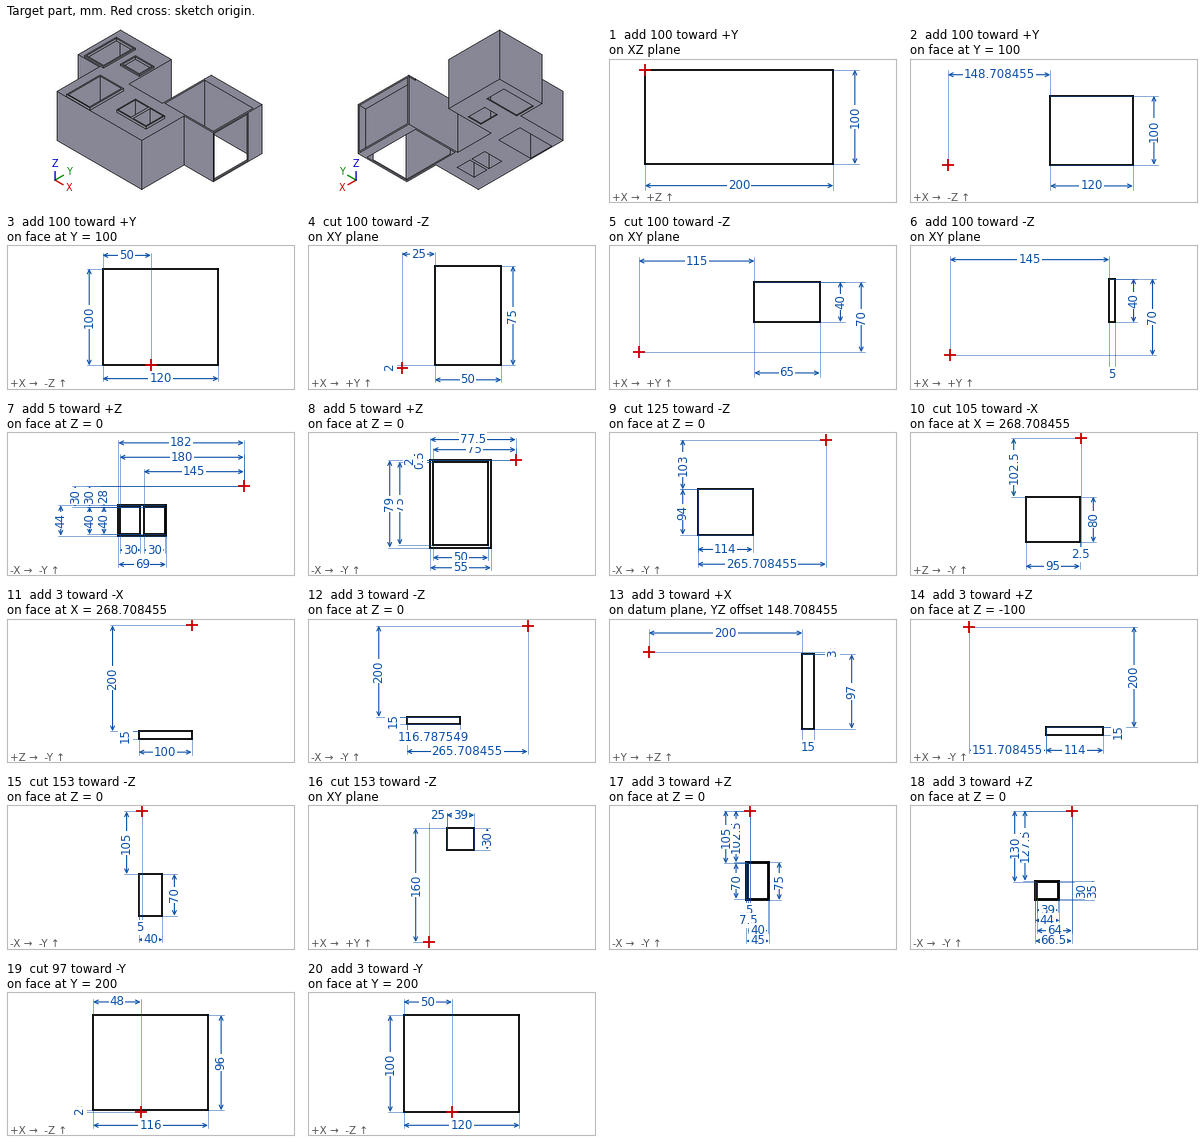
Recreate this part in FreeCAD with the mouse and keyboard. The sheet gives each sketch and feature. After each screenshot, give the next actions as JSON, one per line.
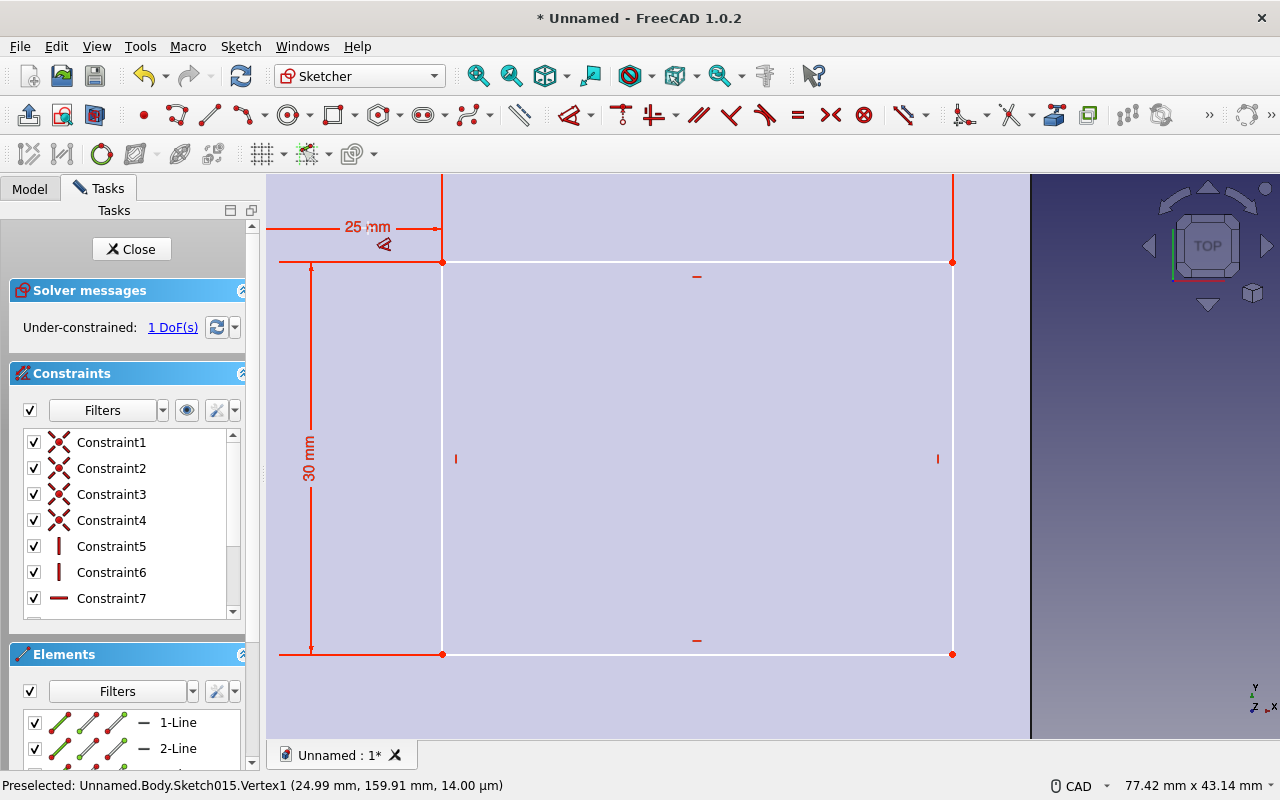
{"action": "left_click", "coordinate": [442, 262]}
{"action": "left_click", "coordinate": [476, 487]}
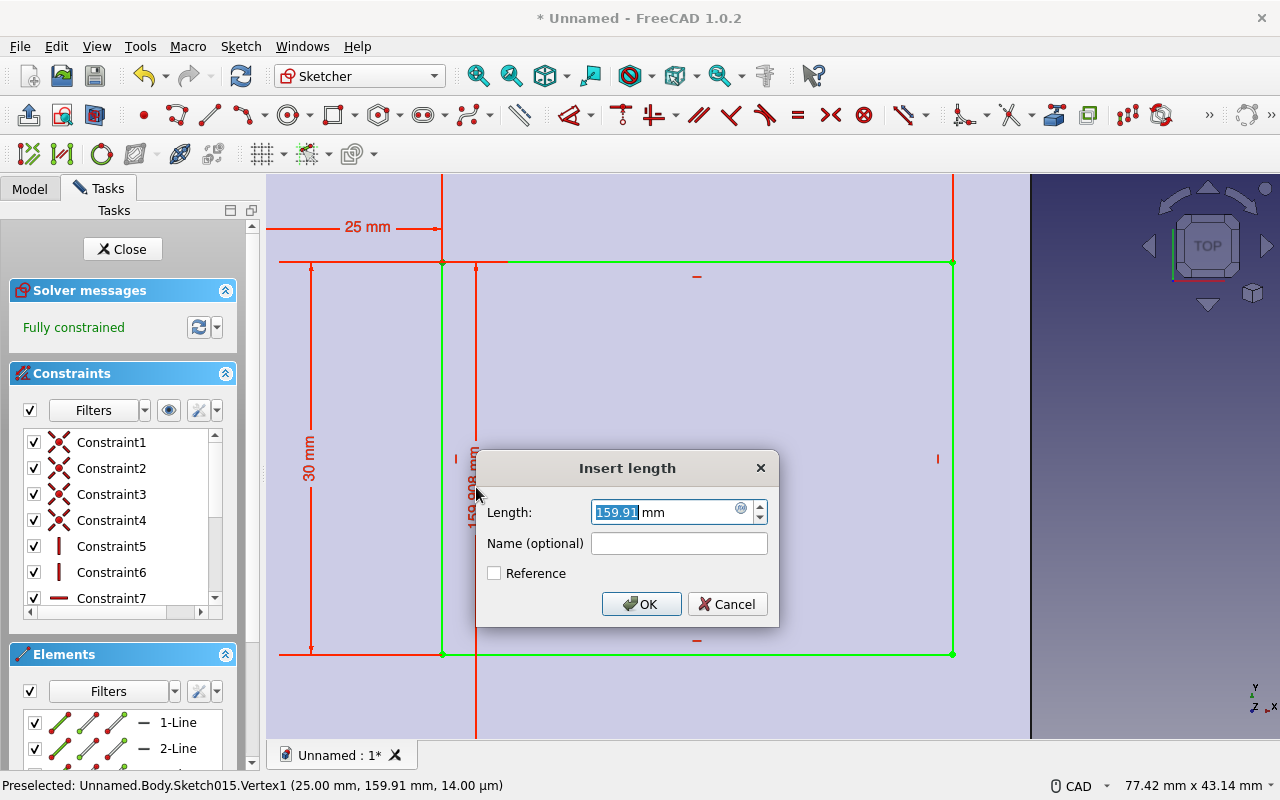
{"action": "type", "text": "160"}
{"action": "key", "text": "Return"}
{"action": "key", "text": "Escape"}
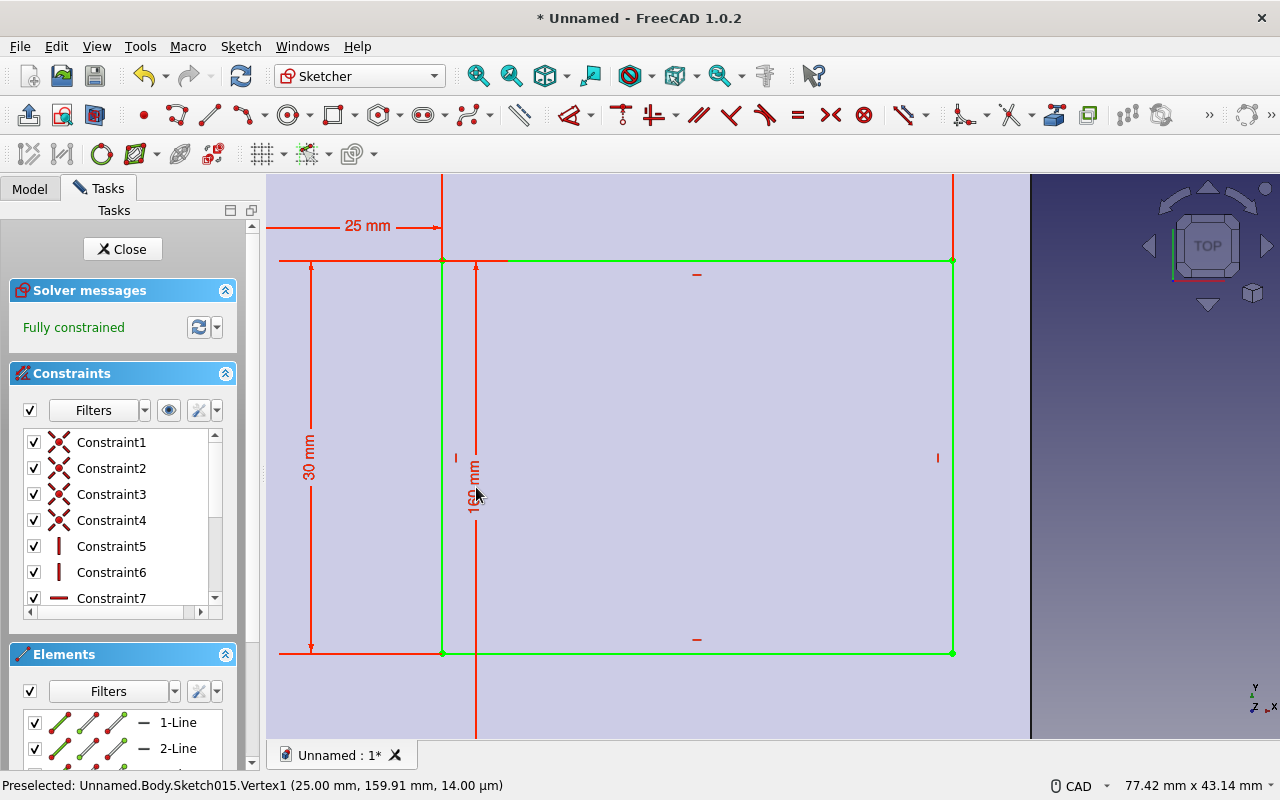
{"action": "left_click", "coordinate": [123, 249]}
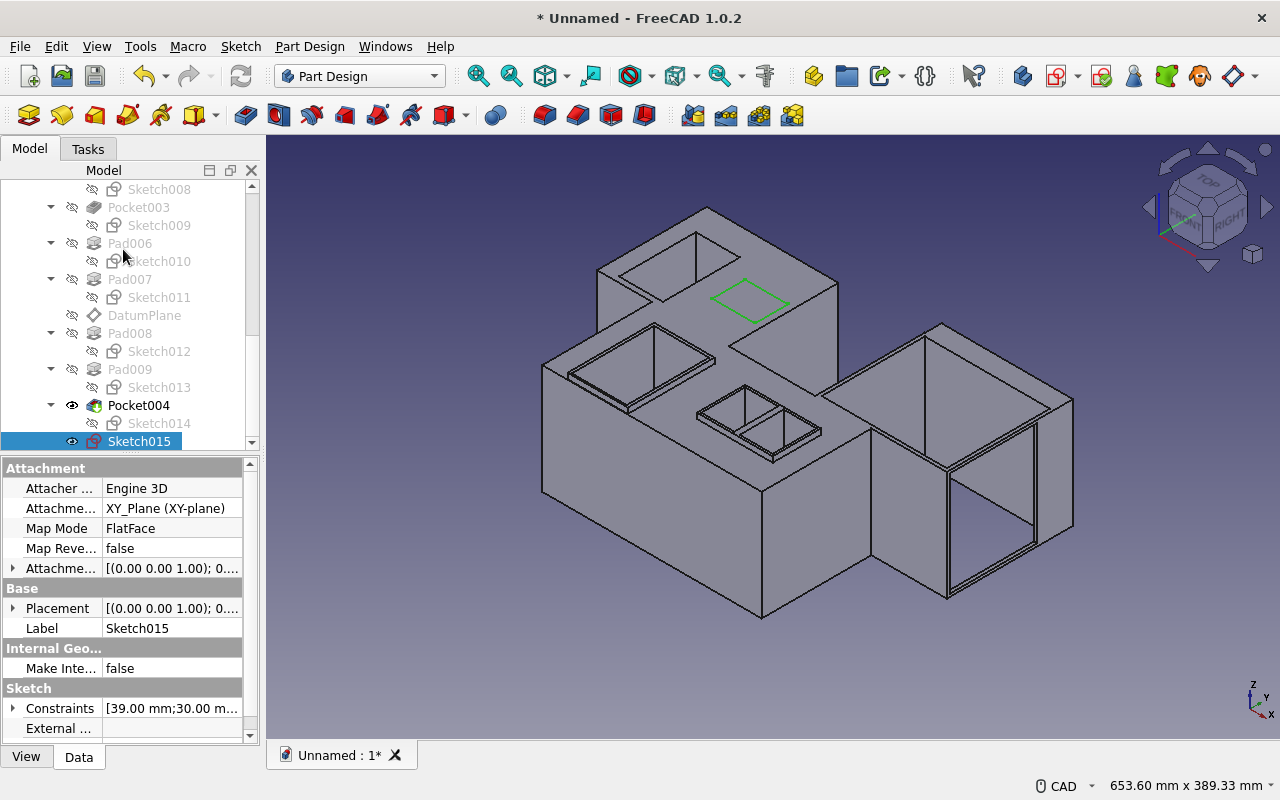
{"action": "left_click", "coordinate": [246, 116]}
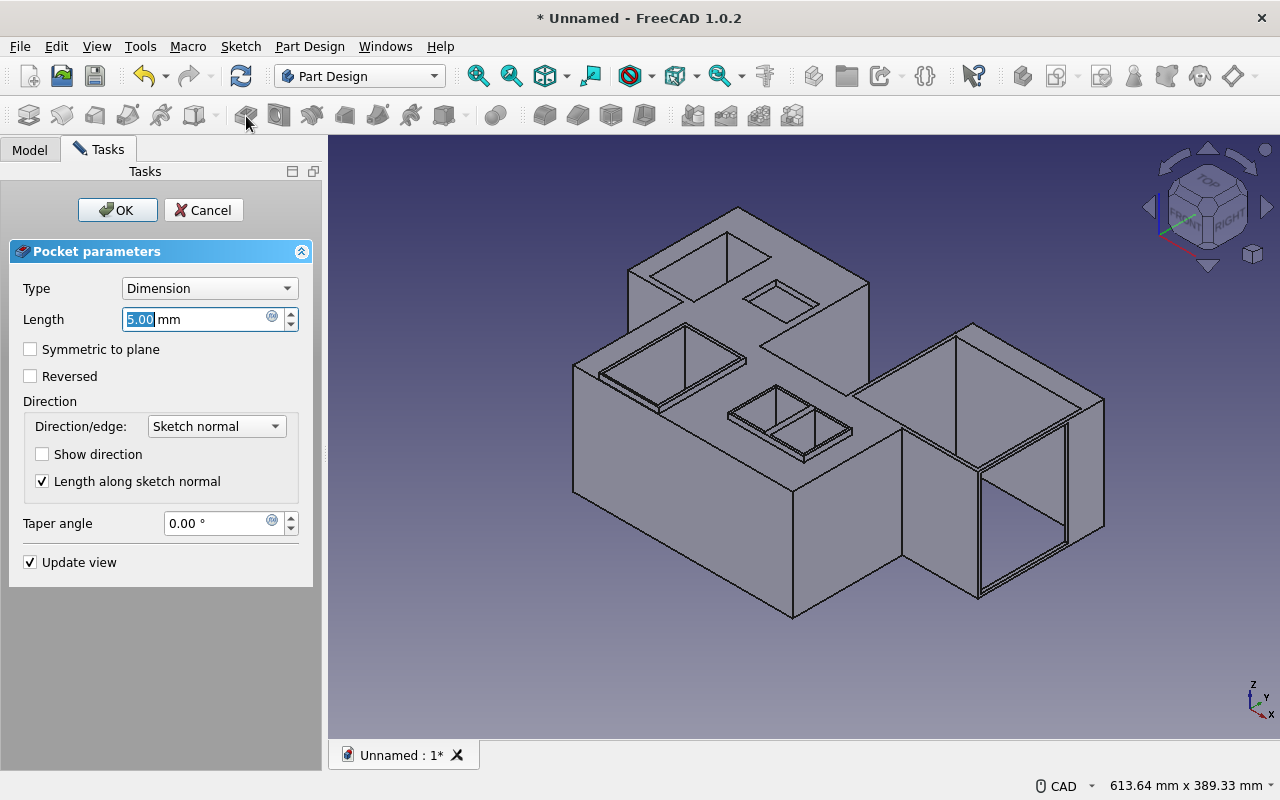
{"action": "type", "text": "153"}
{"action": "key", "text": "Tab"}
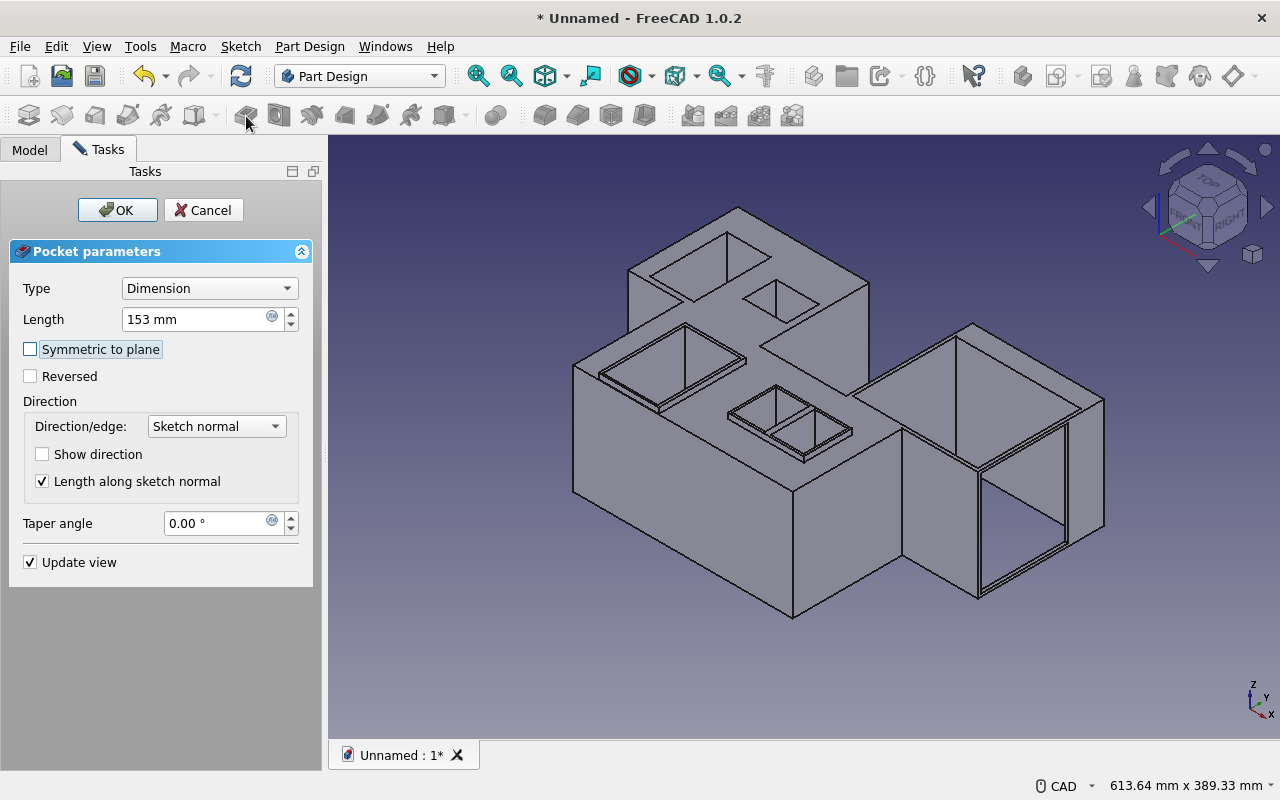
{"action": "left_click", "coordinate": [118, 210]}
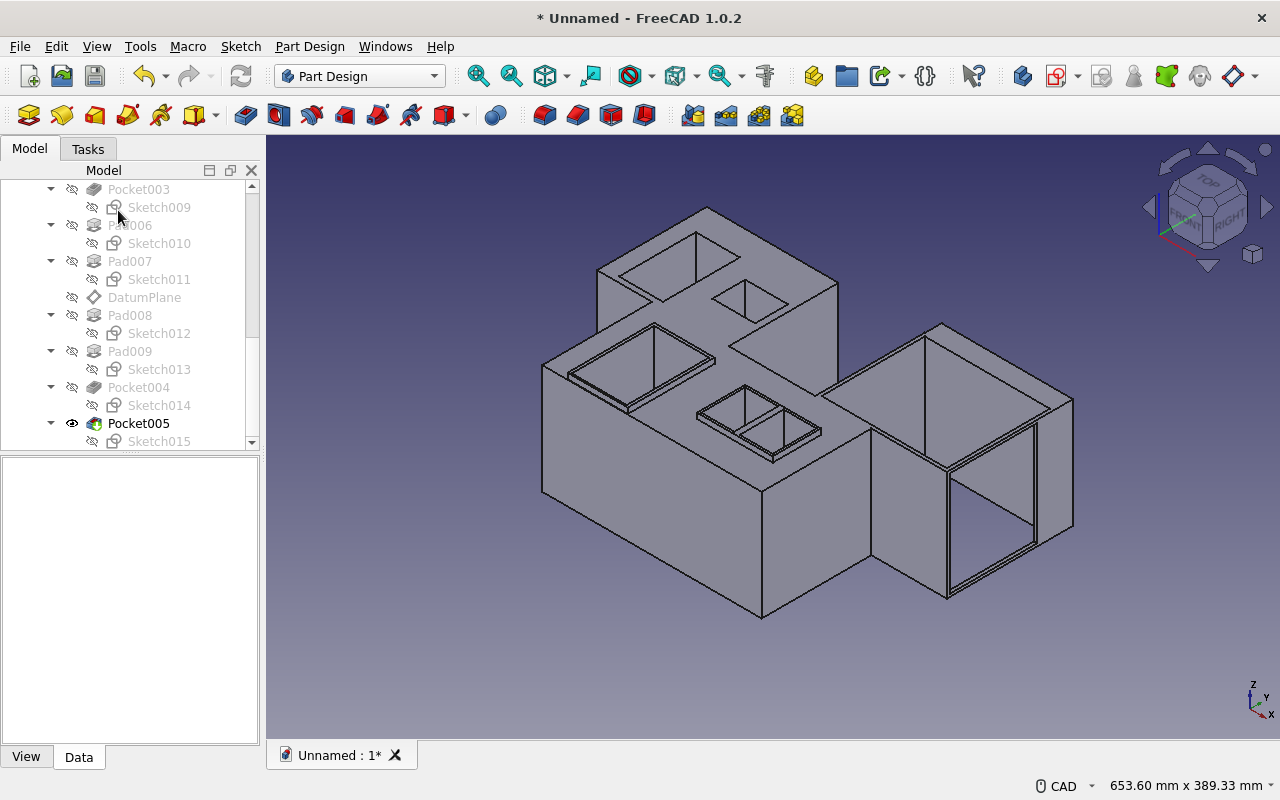
{"action": "left_click", "coordinate": [680, 308]}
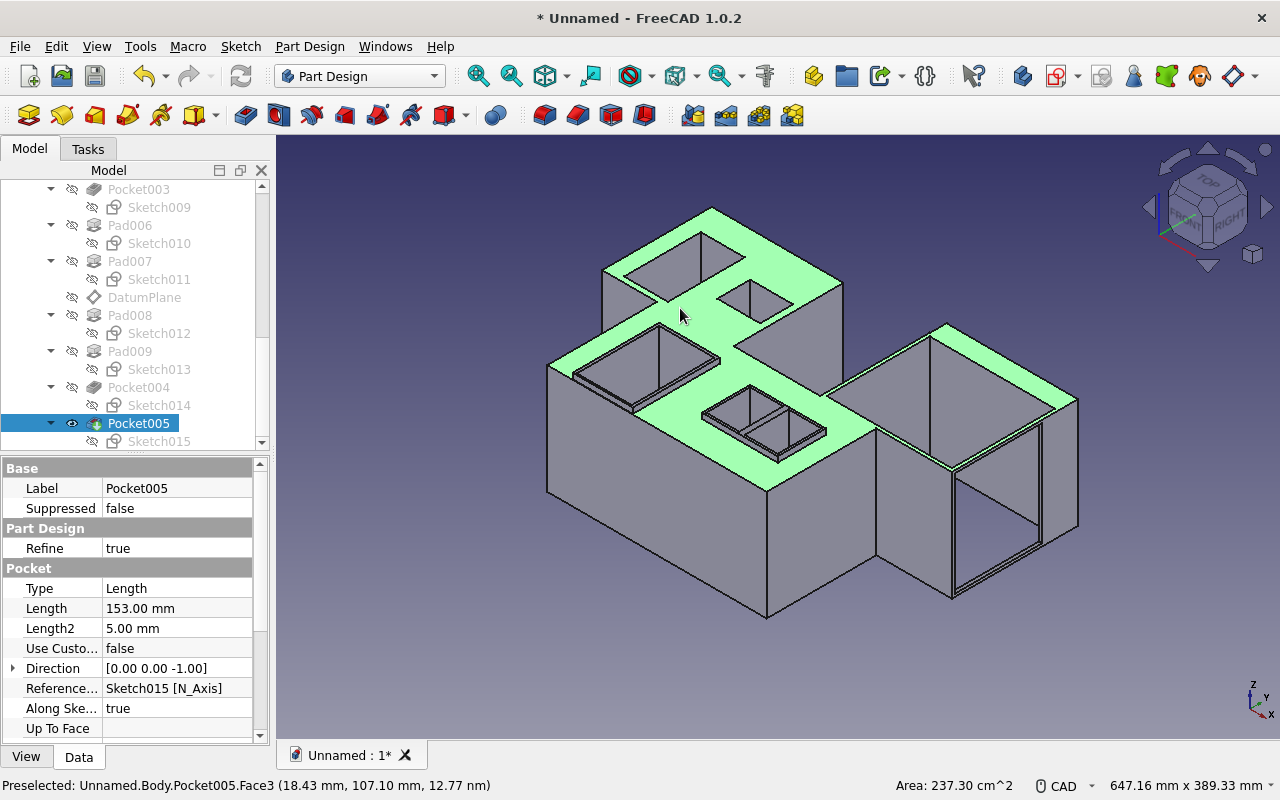
{"action": "left_click", "coordinate": [1056, 76]}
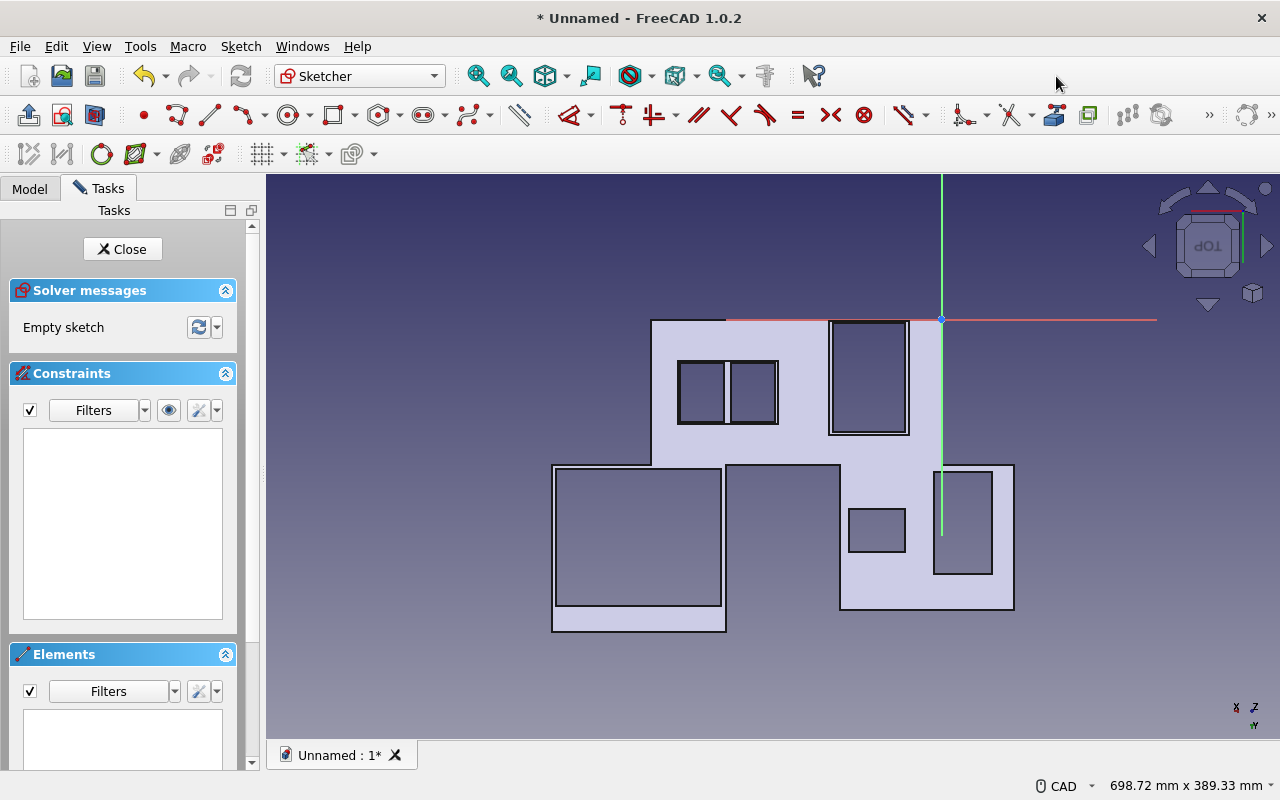
{"action": "scroll", "coordinate": [1115, 433], "scroll_direction": "up", "scroll_amount": 2}